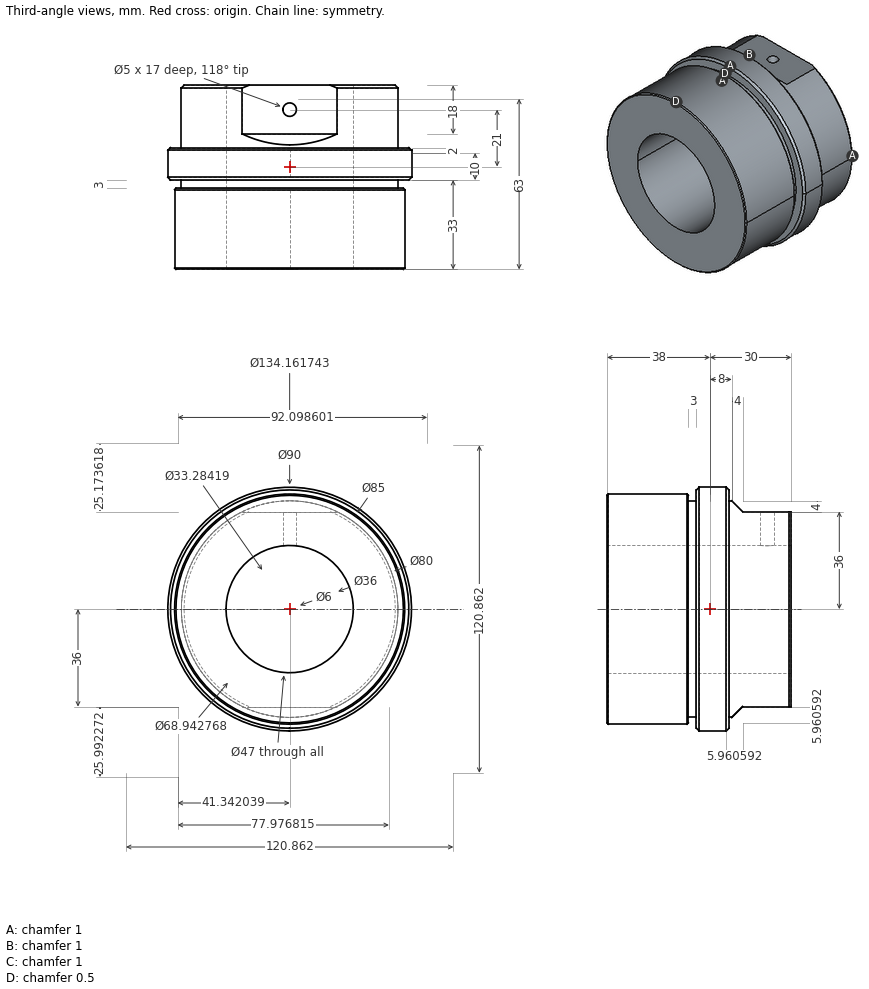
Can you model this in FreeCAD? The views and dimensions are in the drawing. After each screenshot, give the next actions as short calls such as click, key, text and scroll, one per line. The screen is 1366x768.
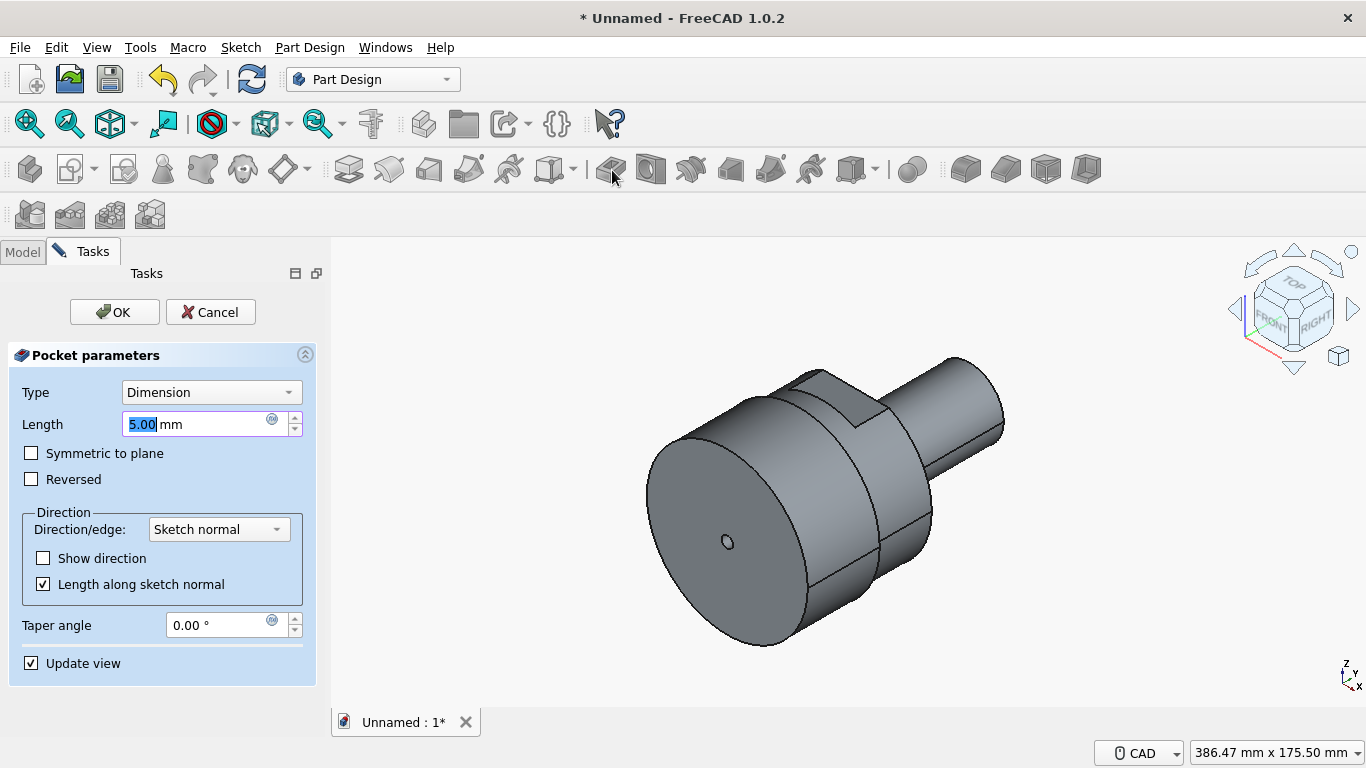
text(63)
key(Tab)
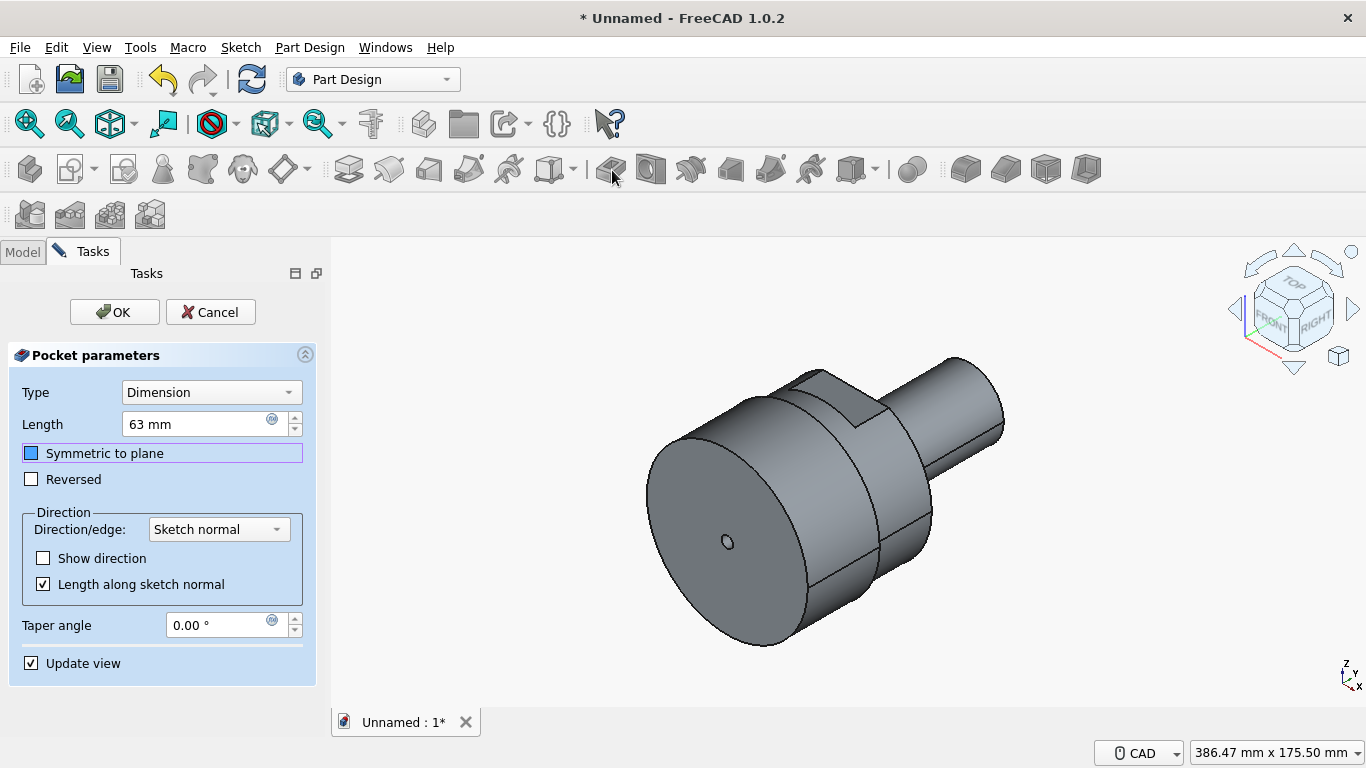
click(115, 312)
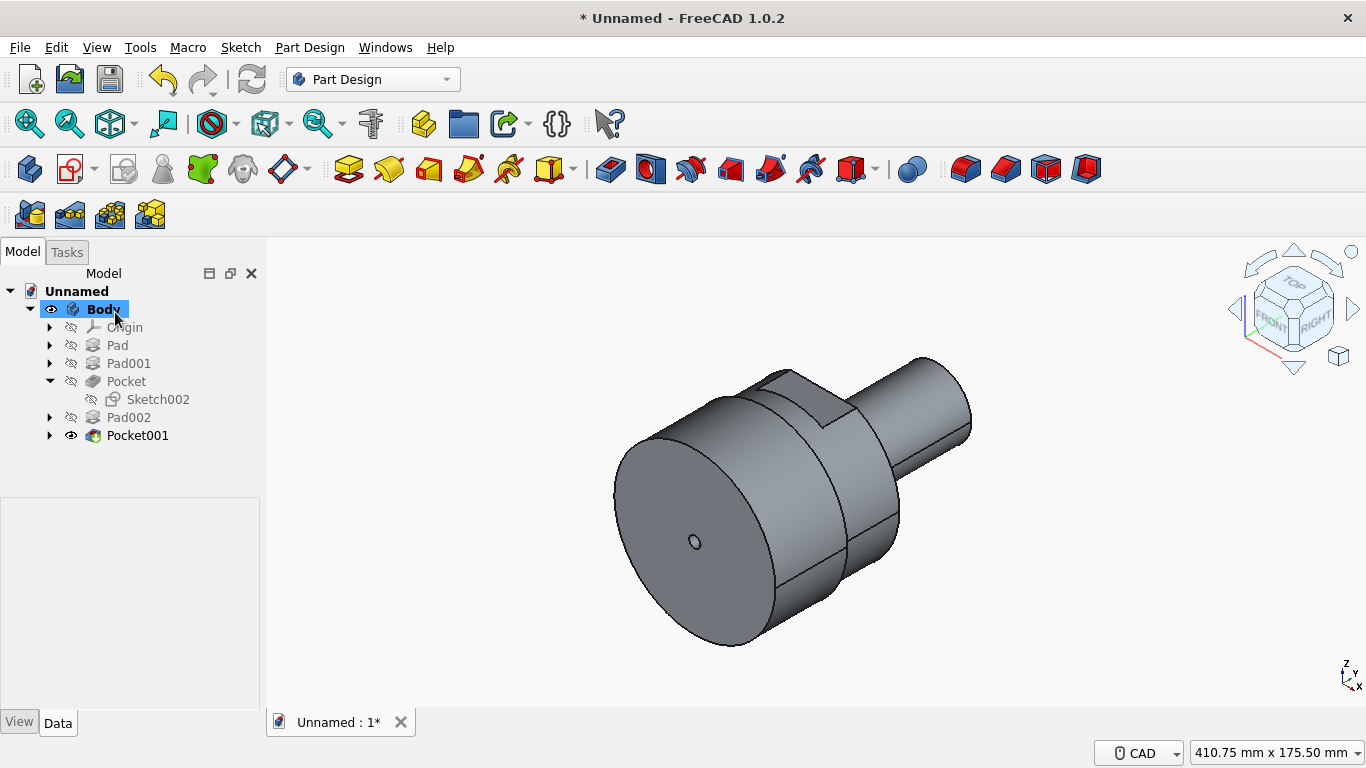
click(50, 327)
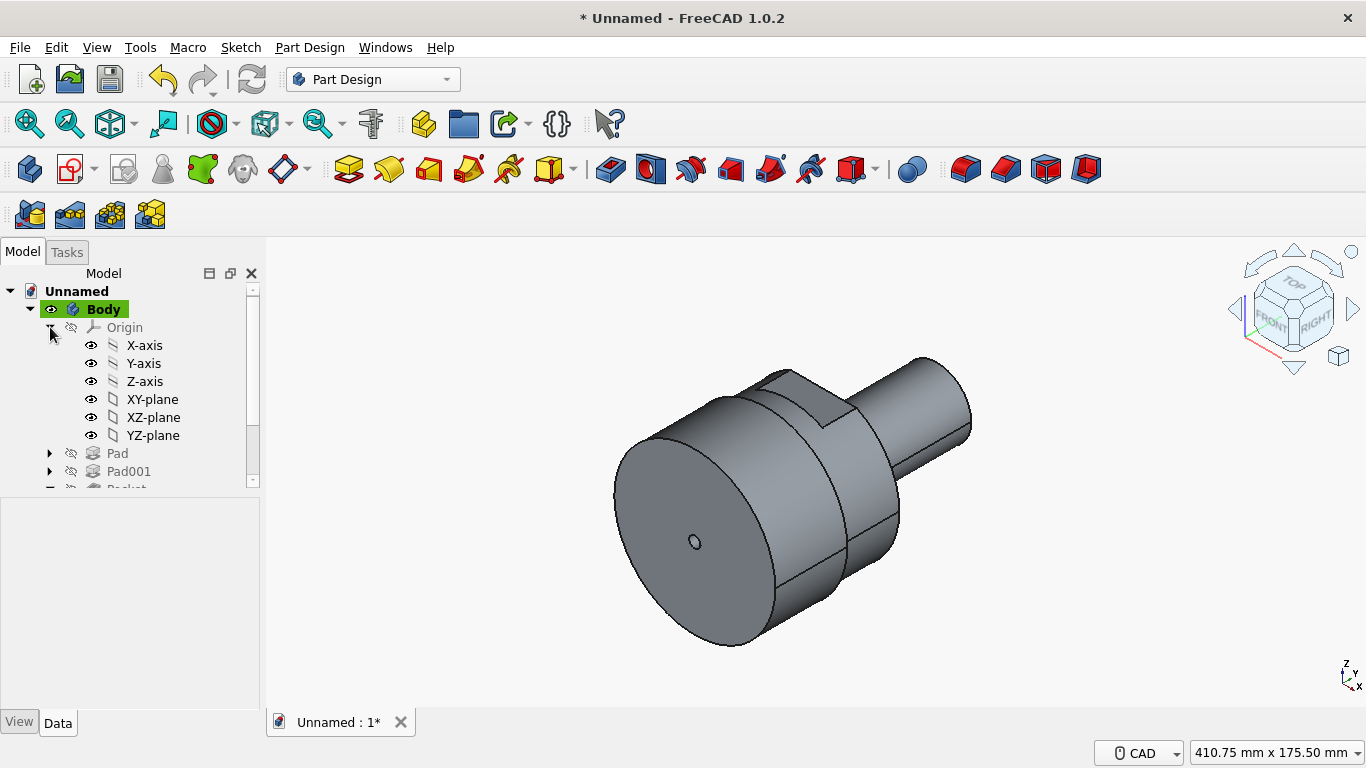
click(136, 417)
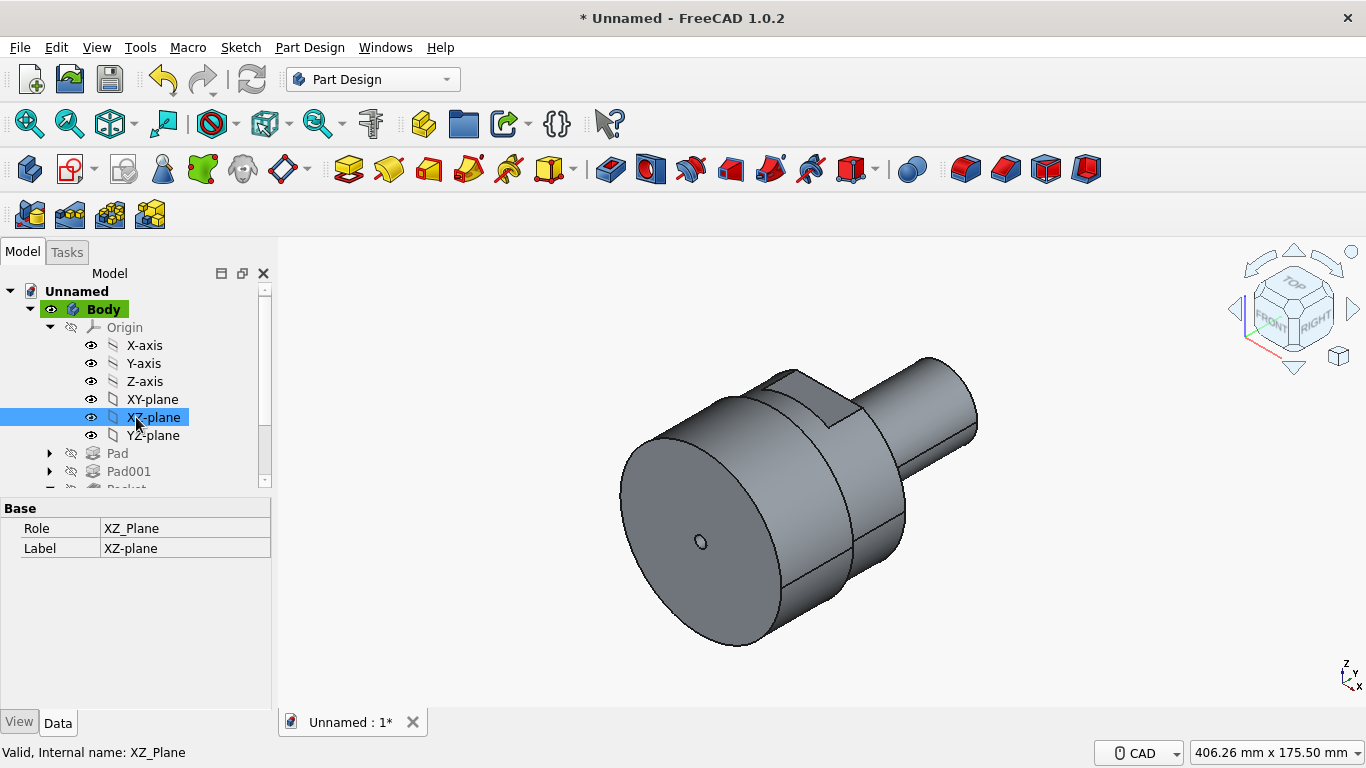
click(284, 170)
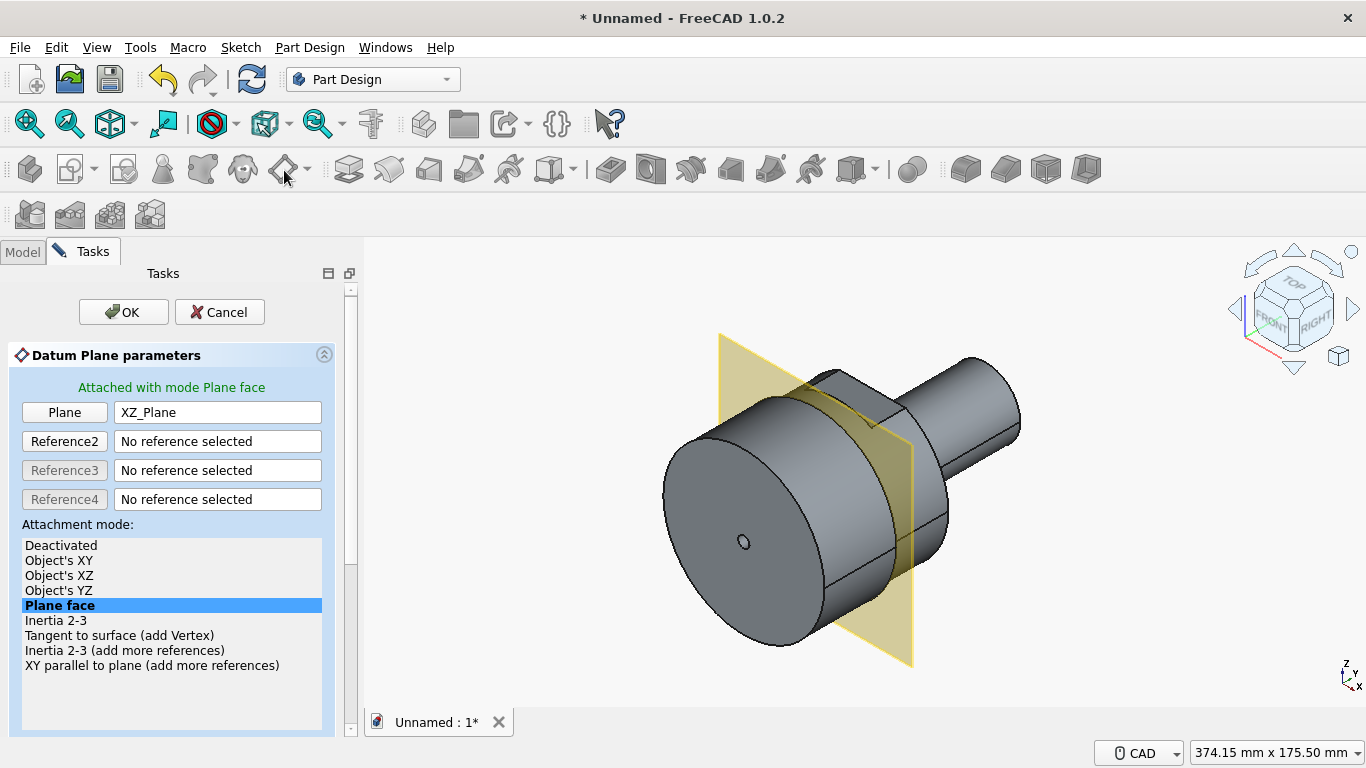
scroll(351, 510, down, 3)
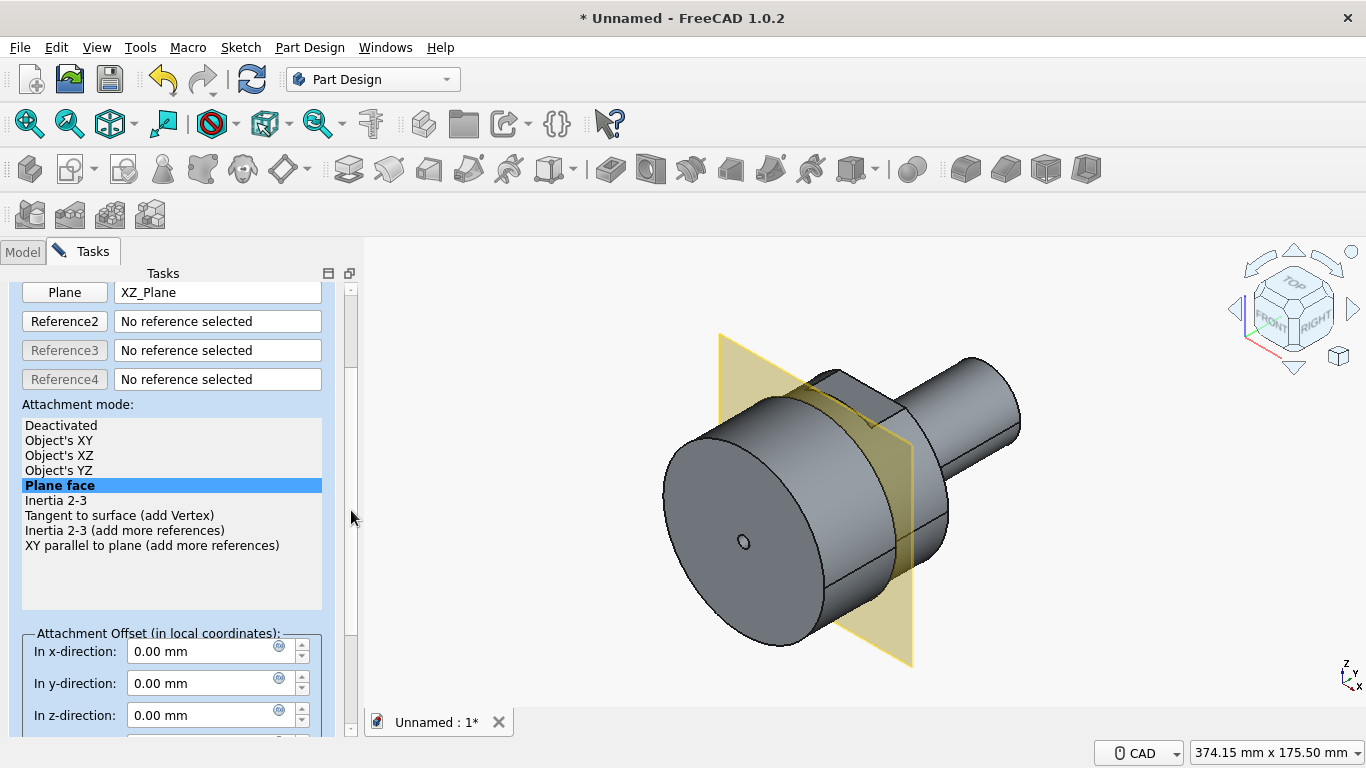
triple_click(210, 655)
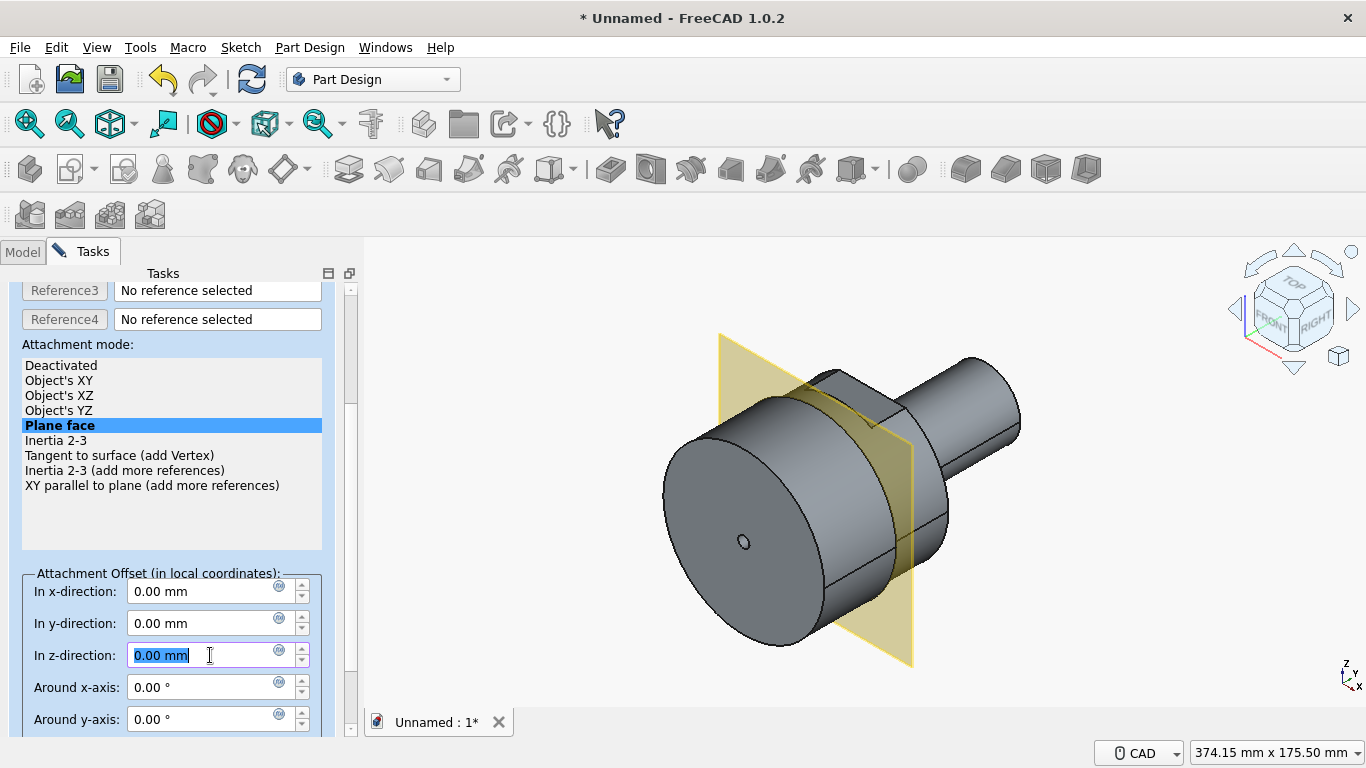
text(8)
key(Tab)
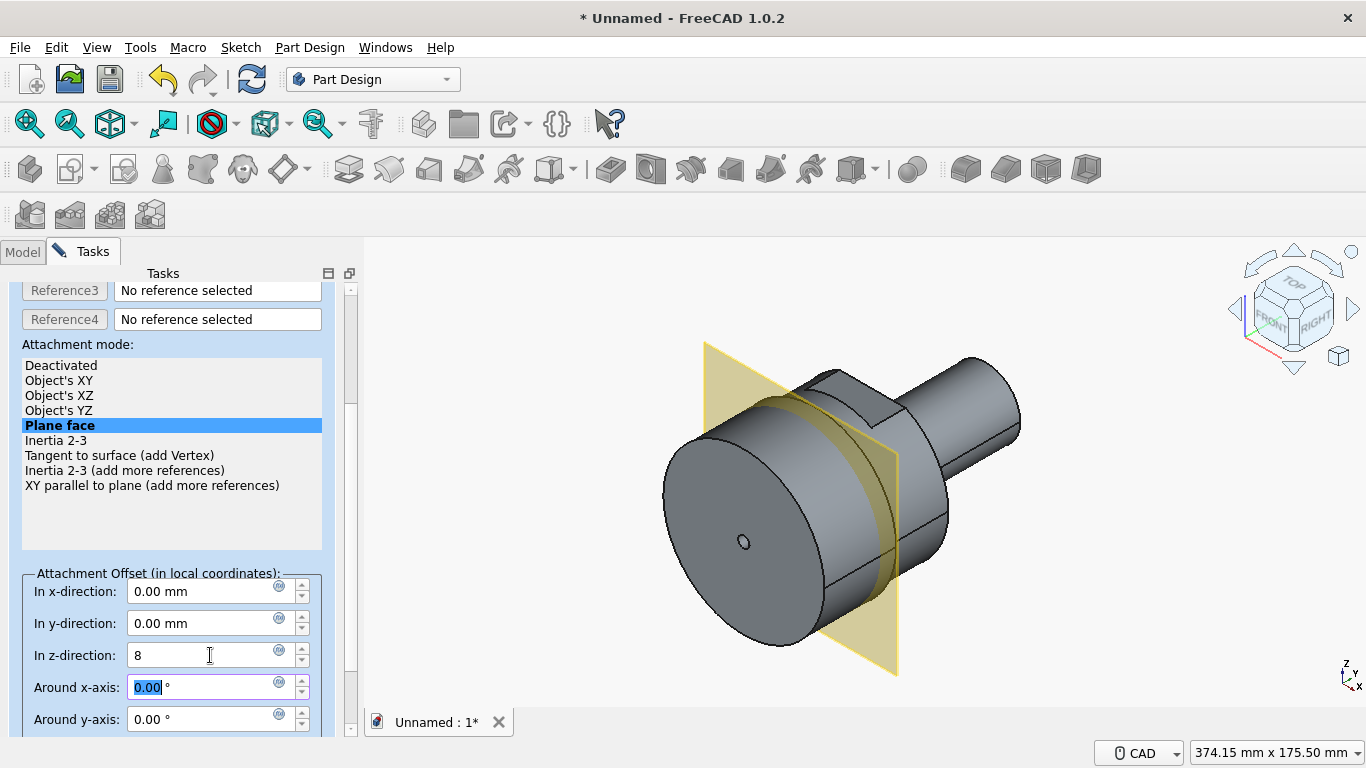
scroll(351, 510, up, 4)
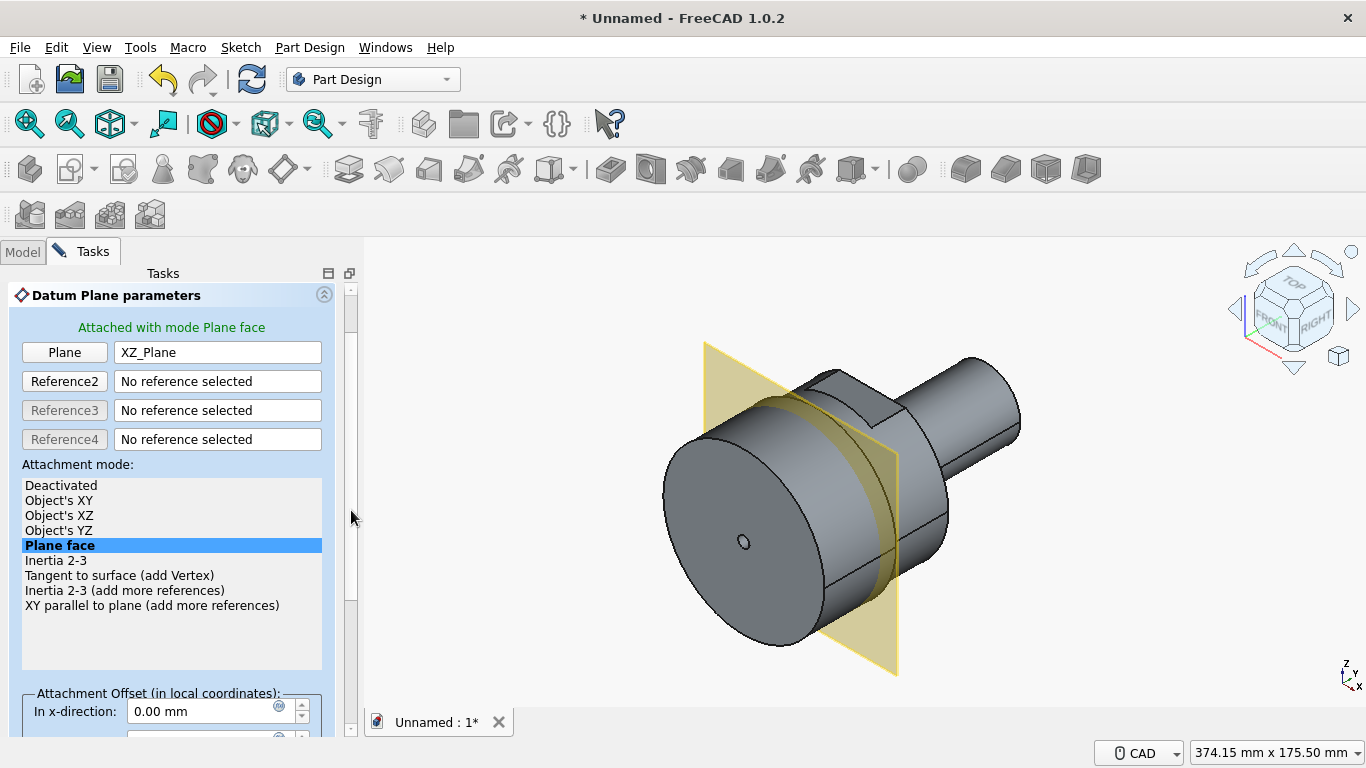
click(124, 312)